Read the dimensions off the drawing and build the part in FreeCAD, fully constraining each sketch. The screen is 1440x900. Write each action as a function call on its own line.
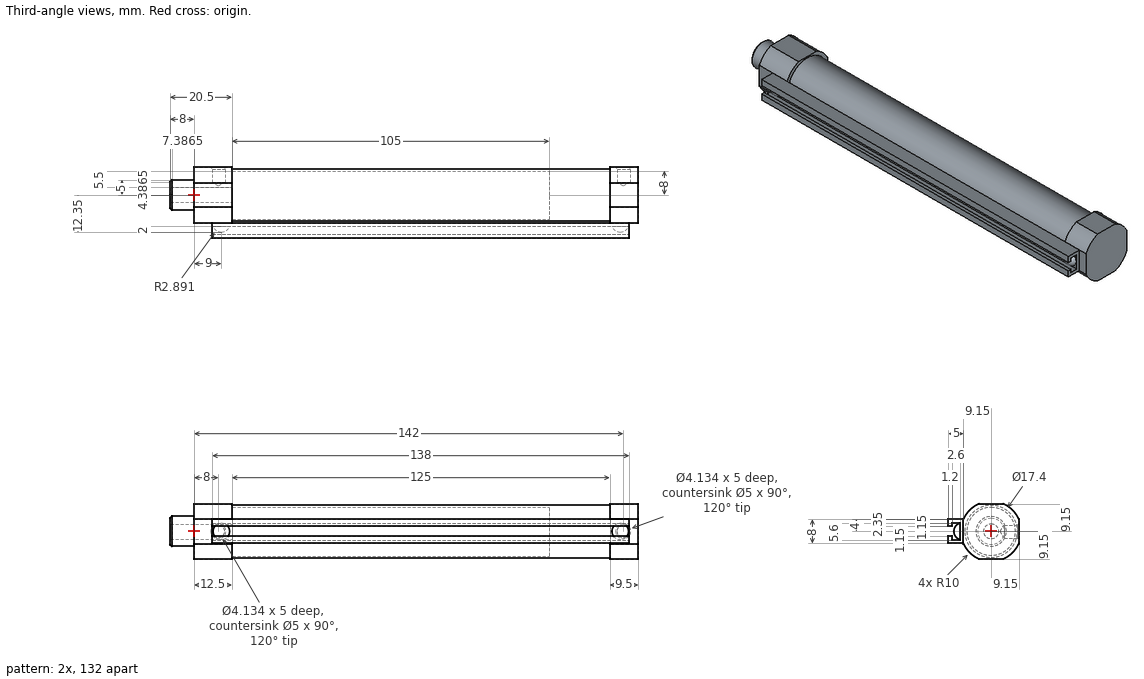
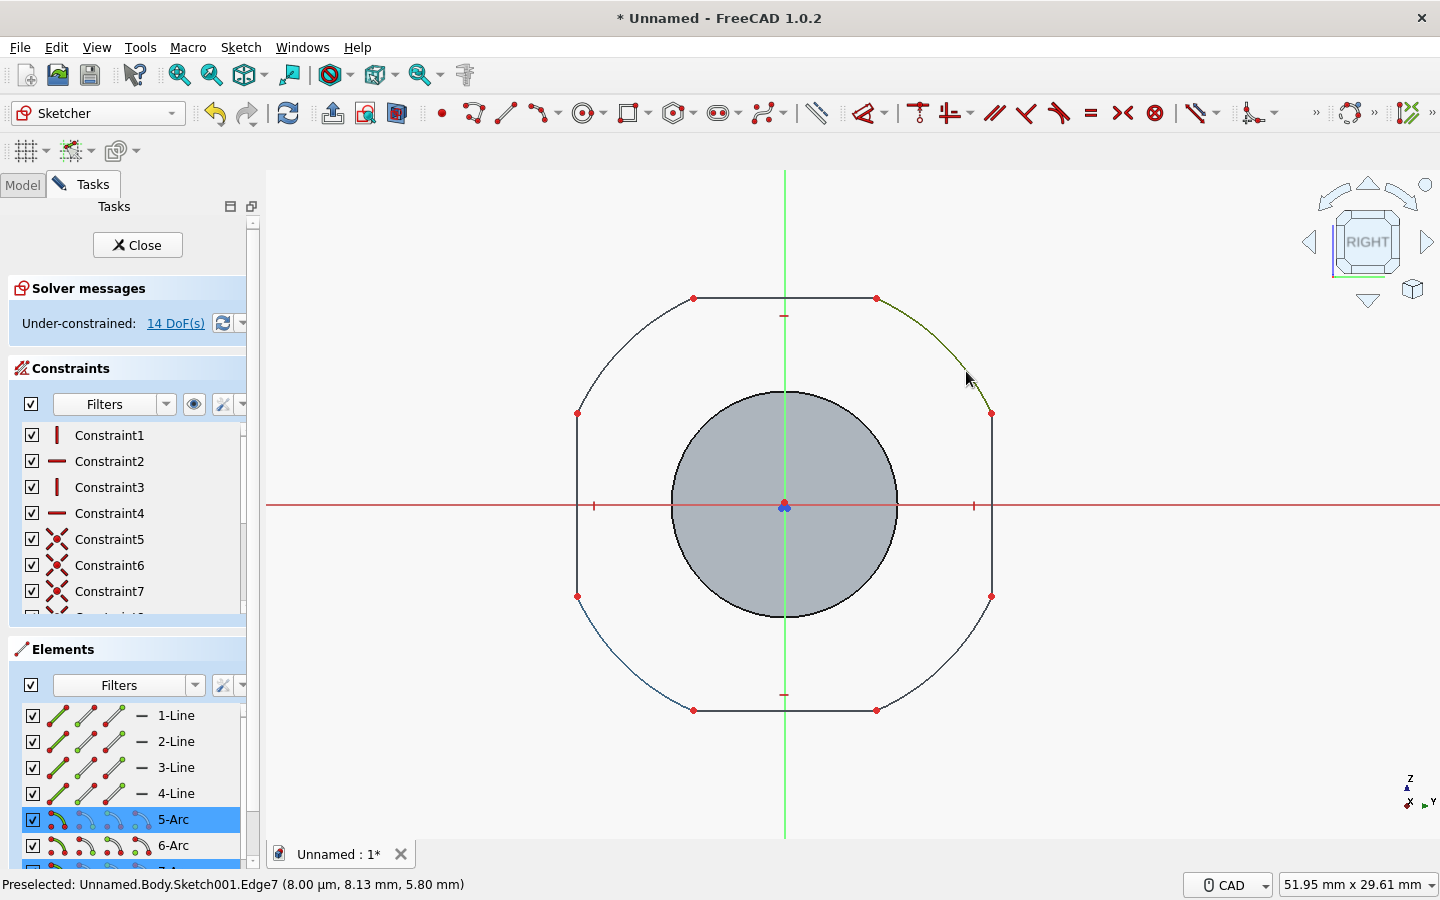
click(918, 114)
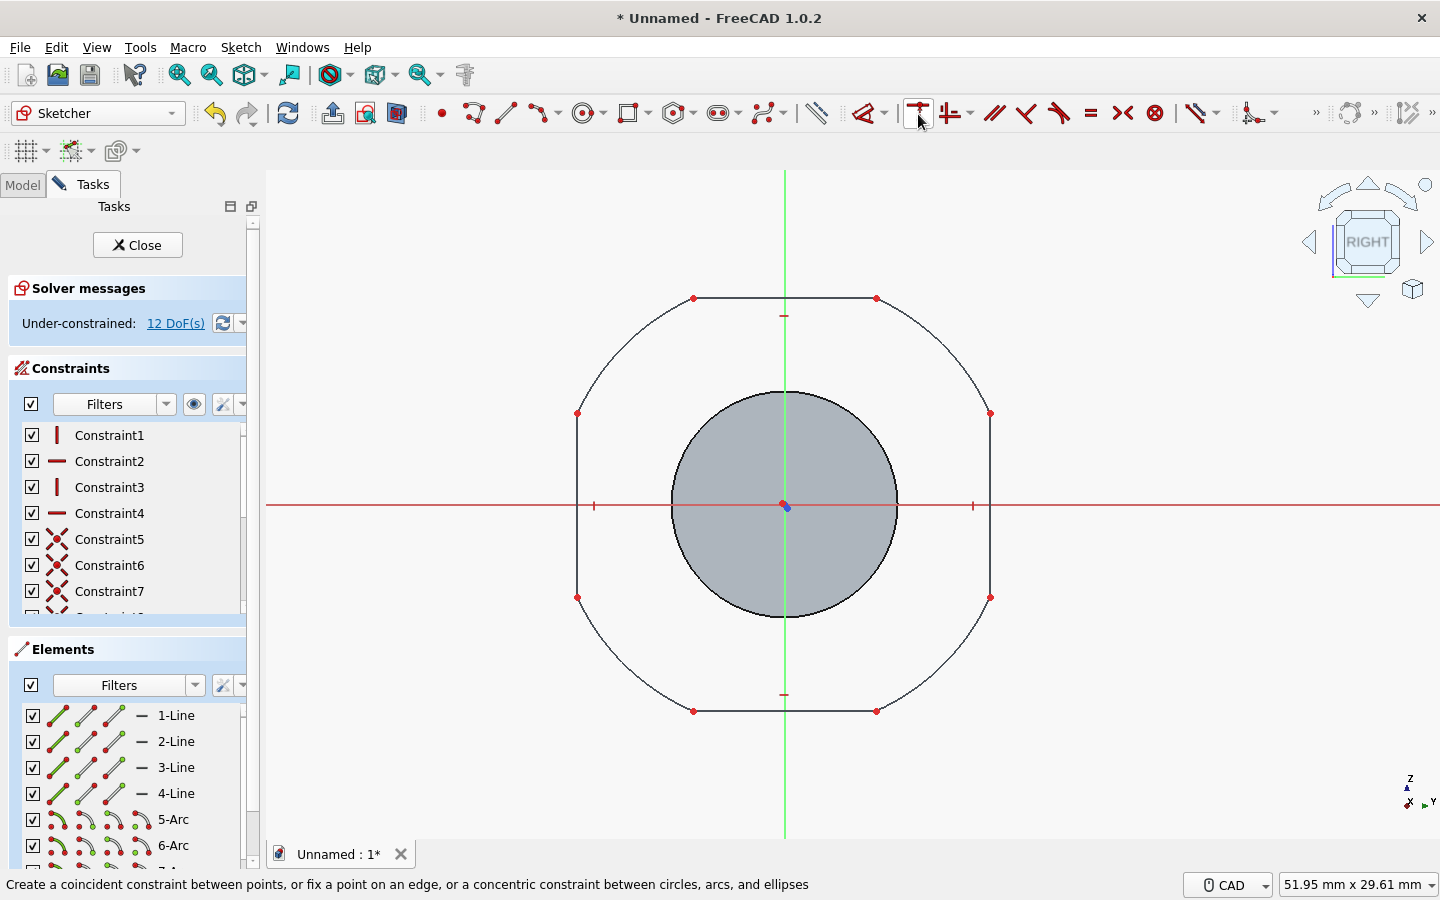
click(603, 640)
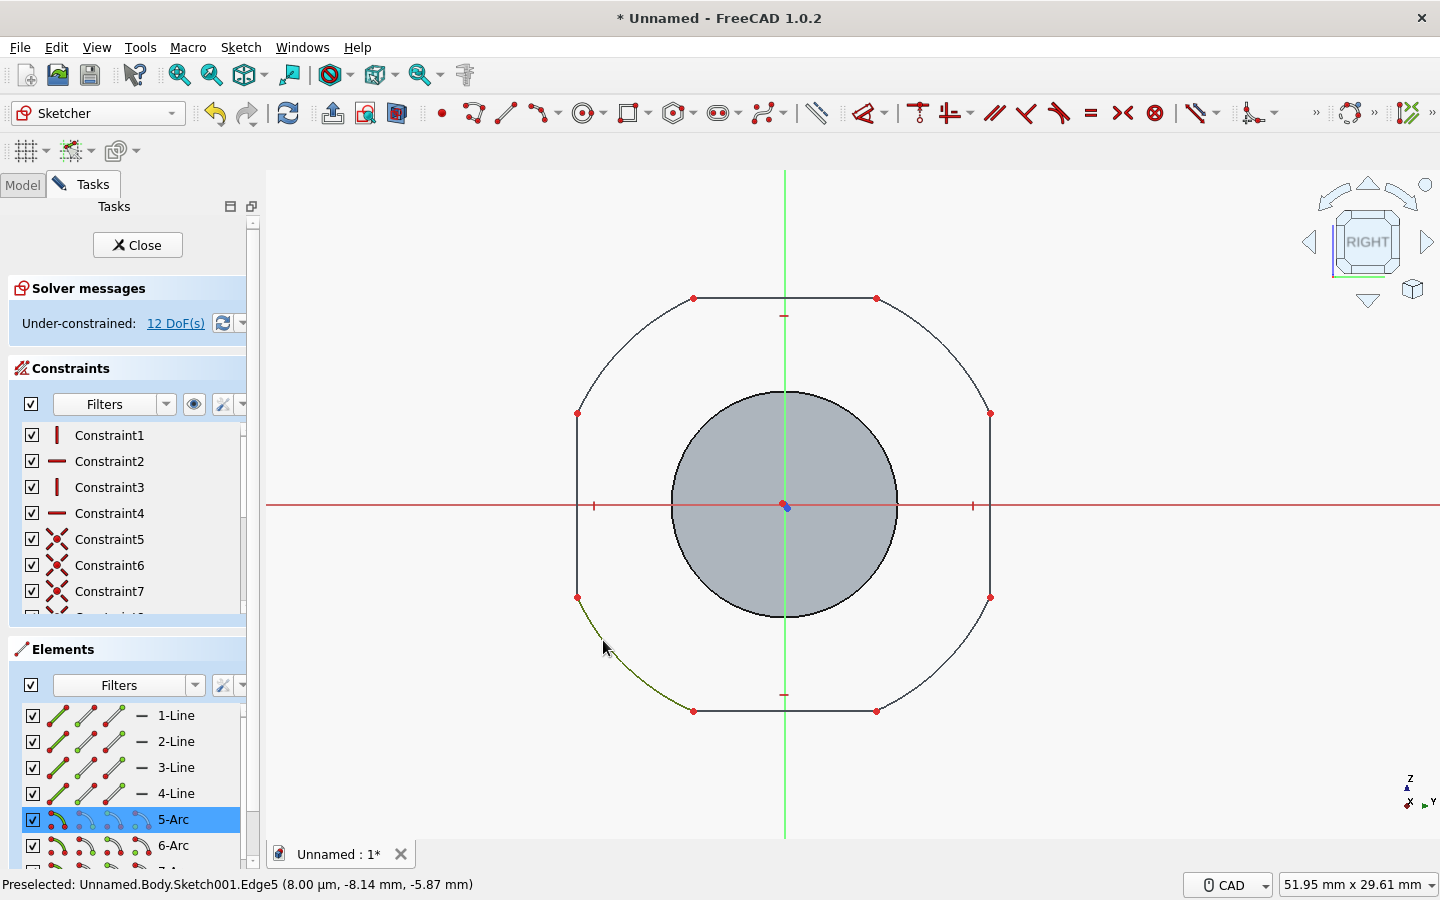
click(650, 324)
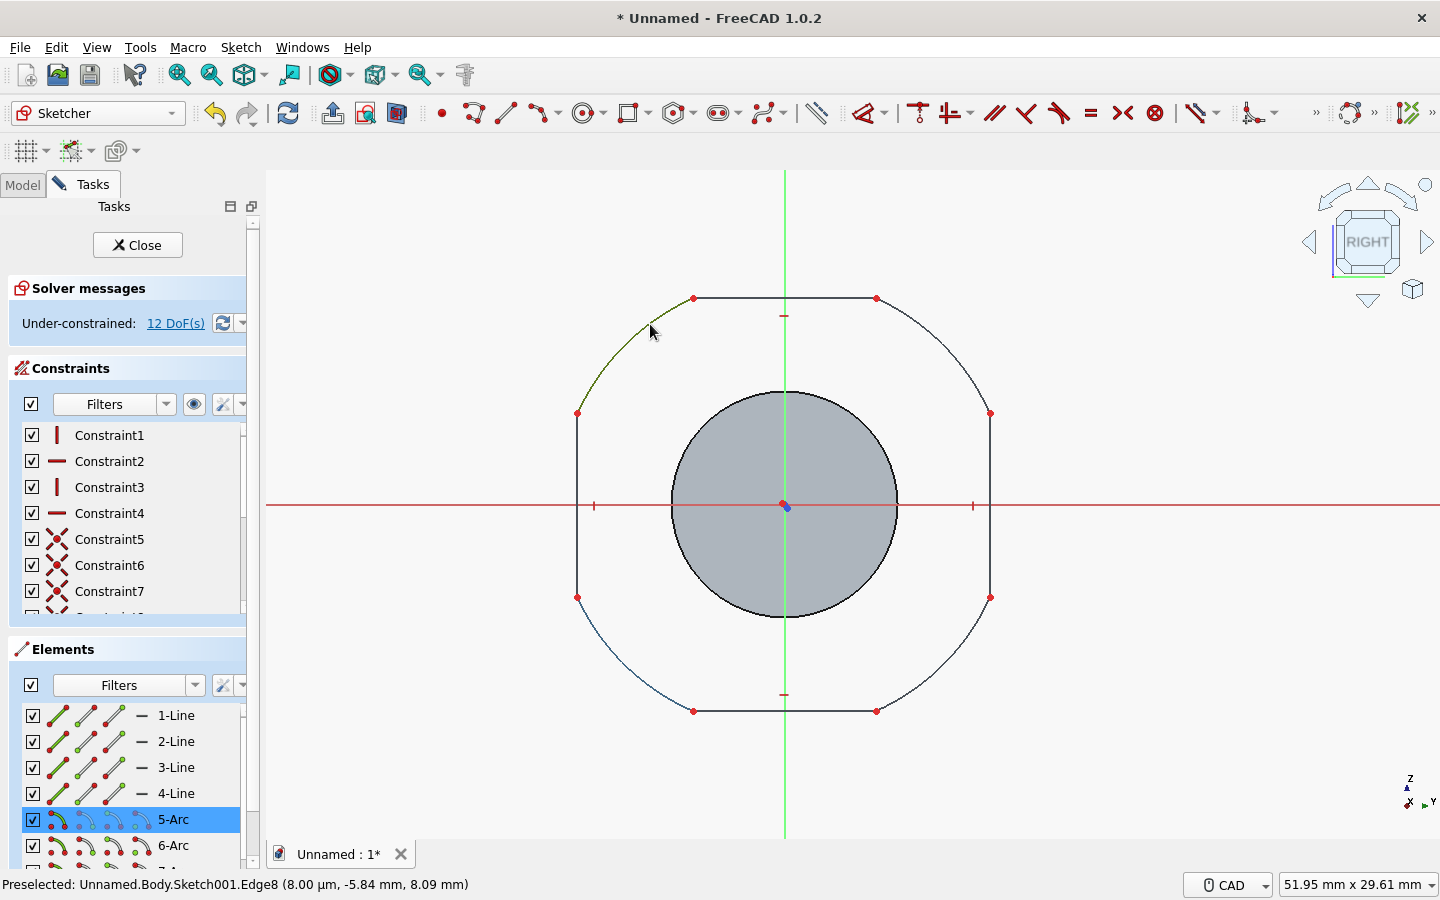
click(918, 114)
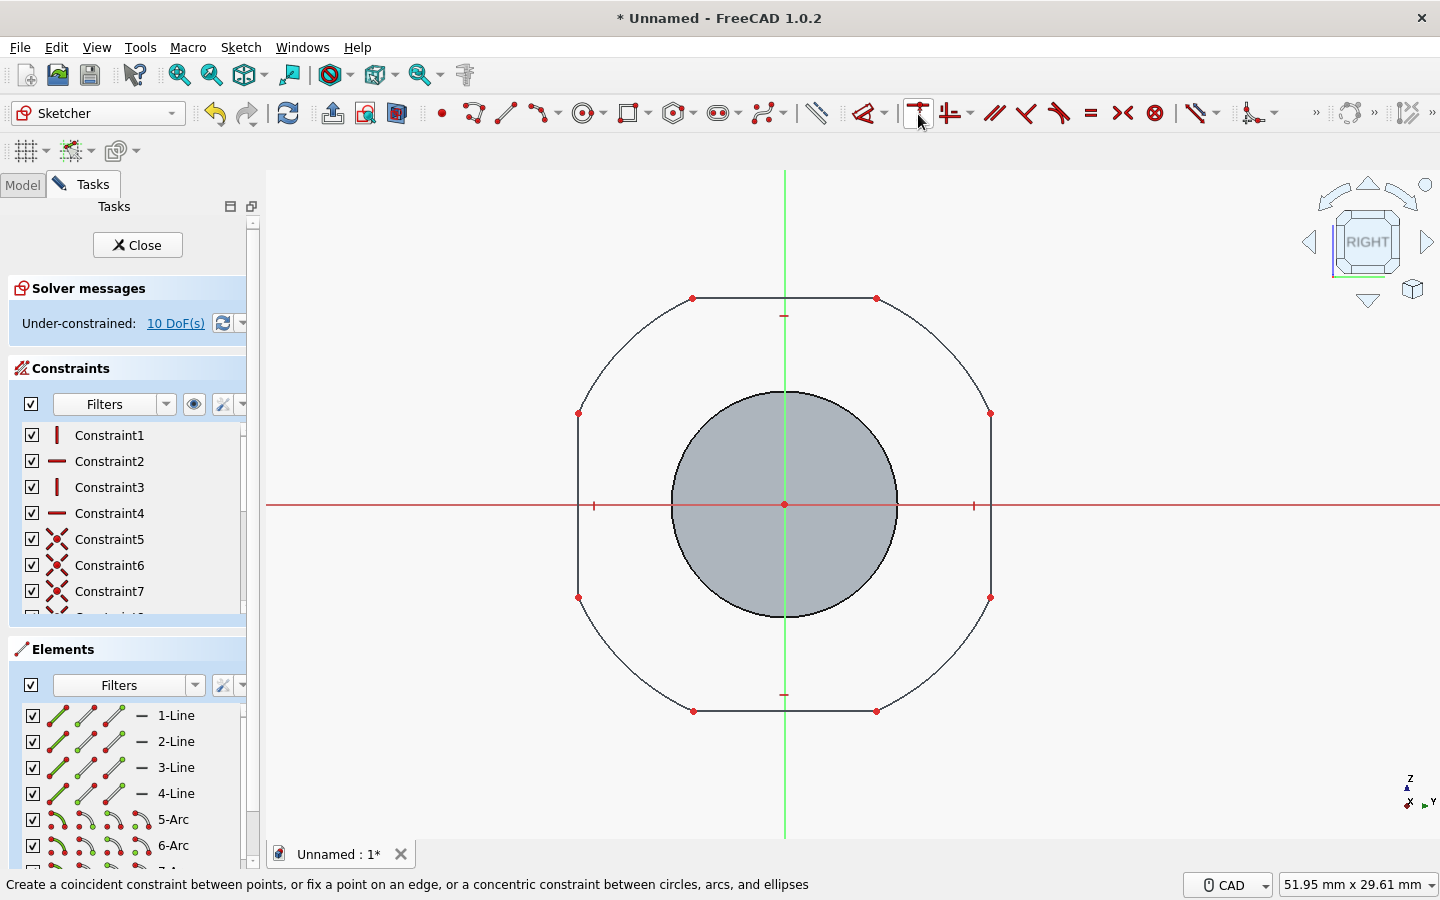
drag(774, 494, 795, 514)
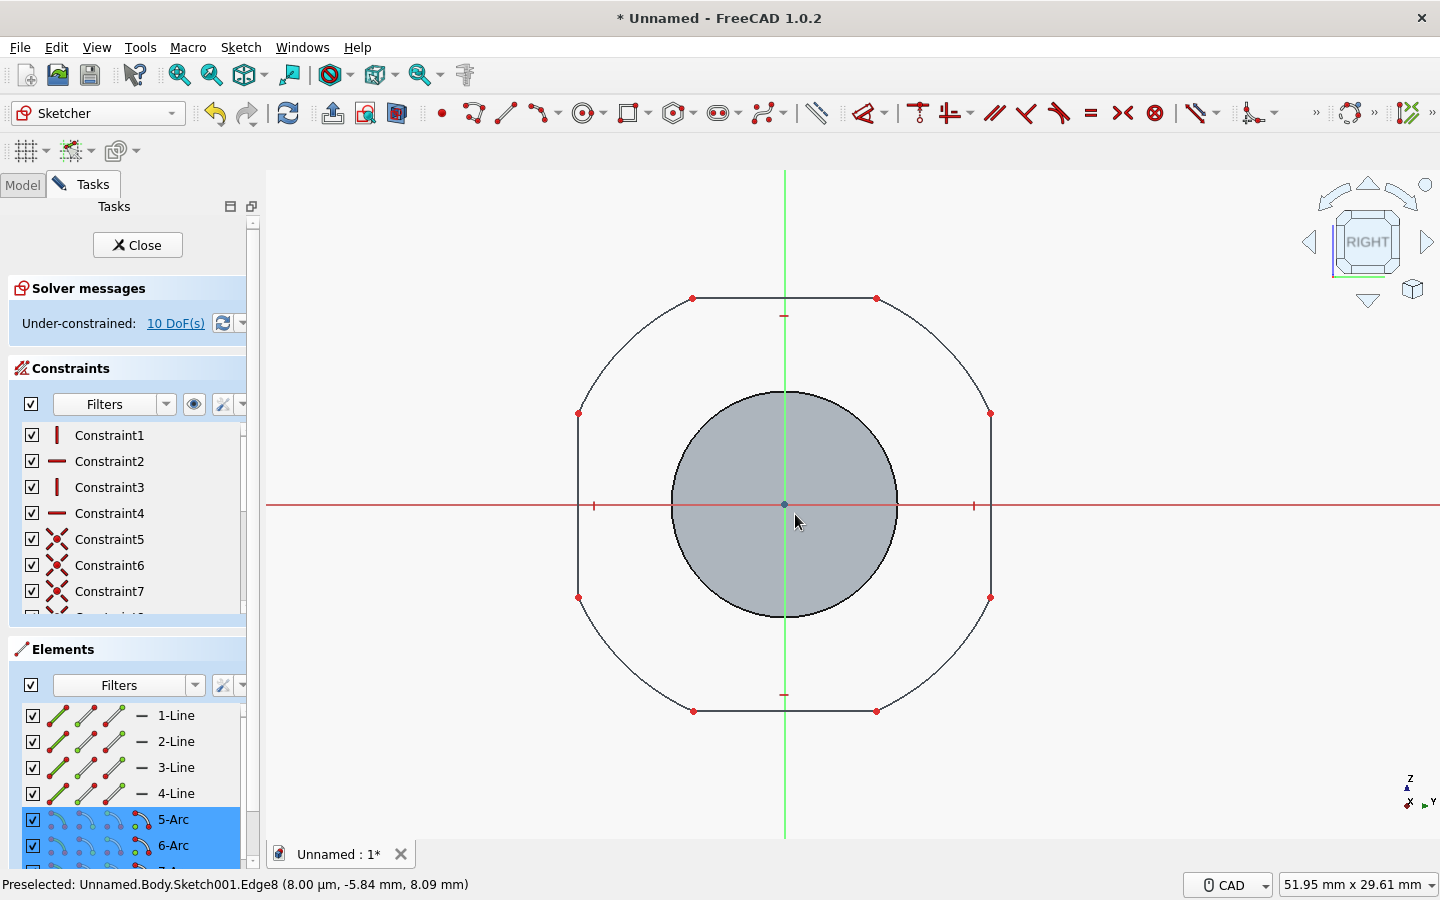
click(918, 114)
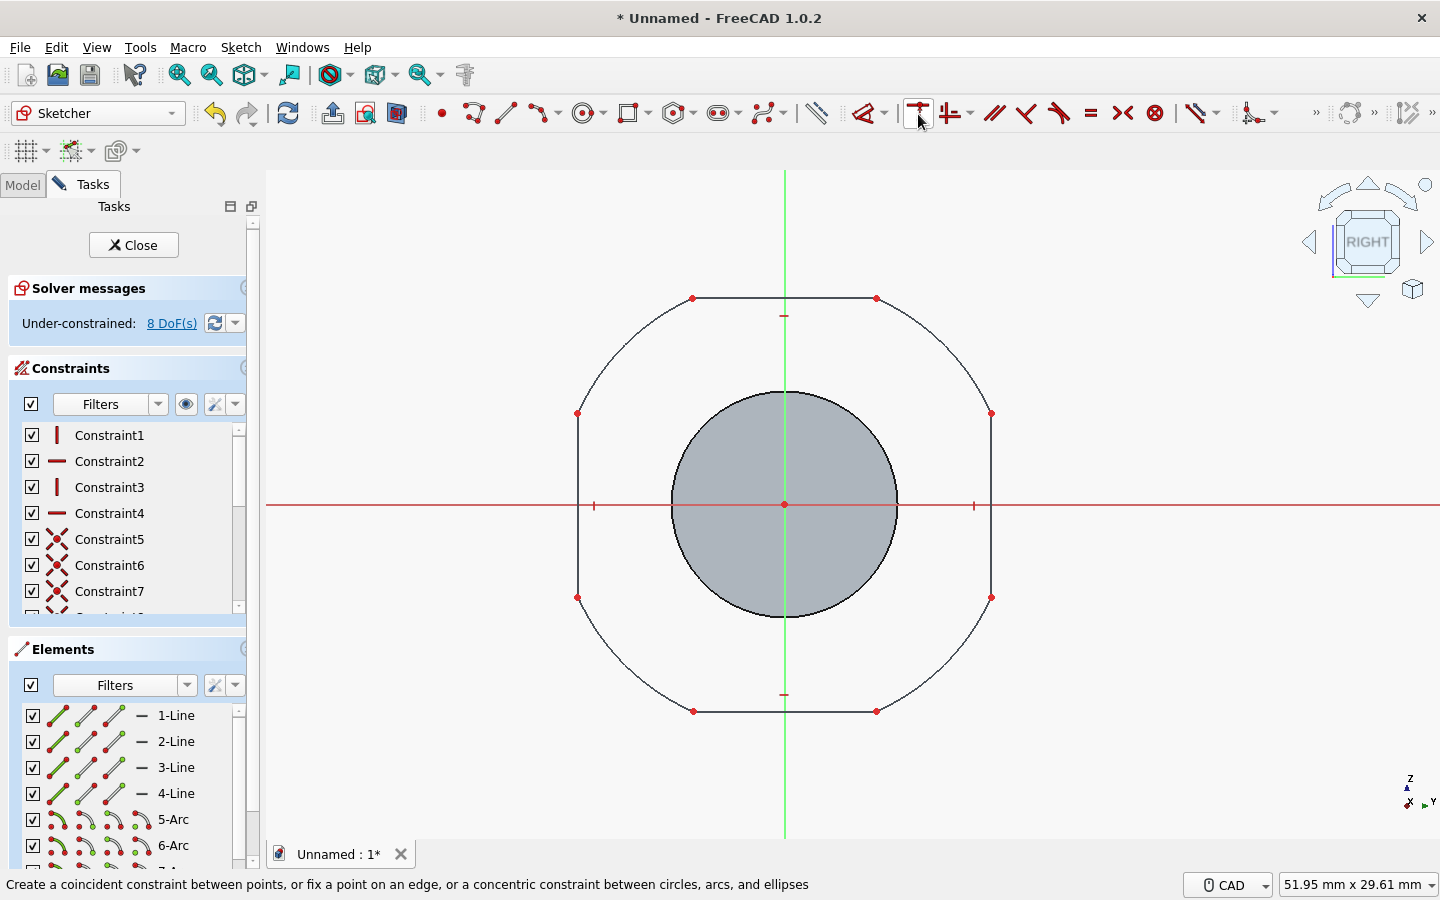
click(603, 640)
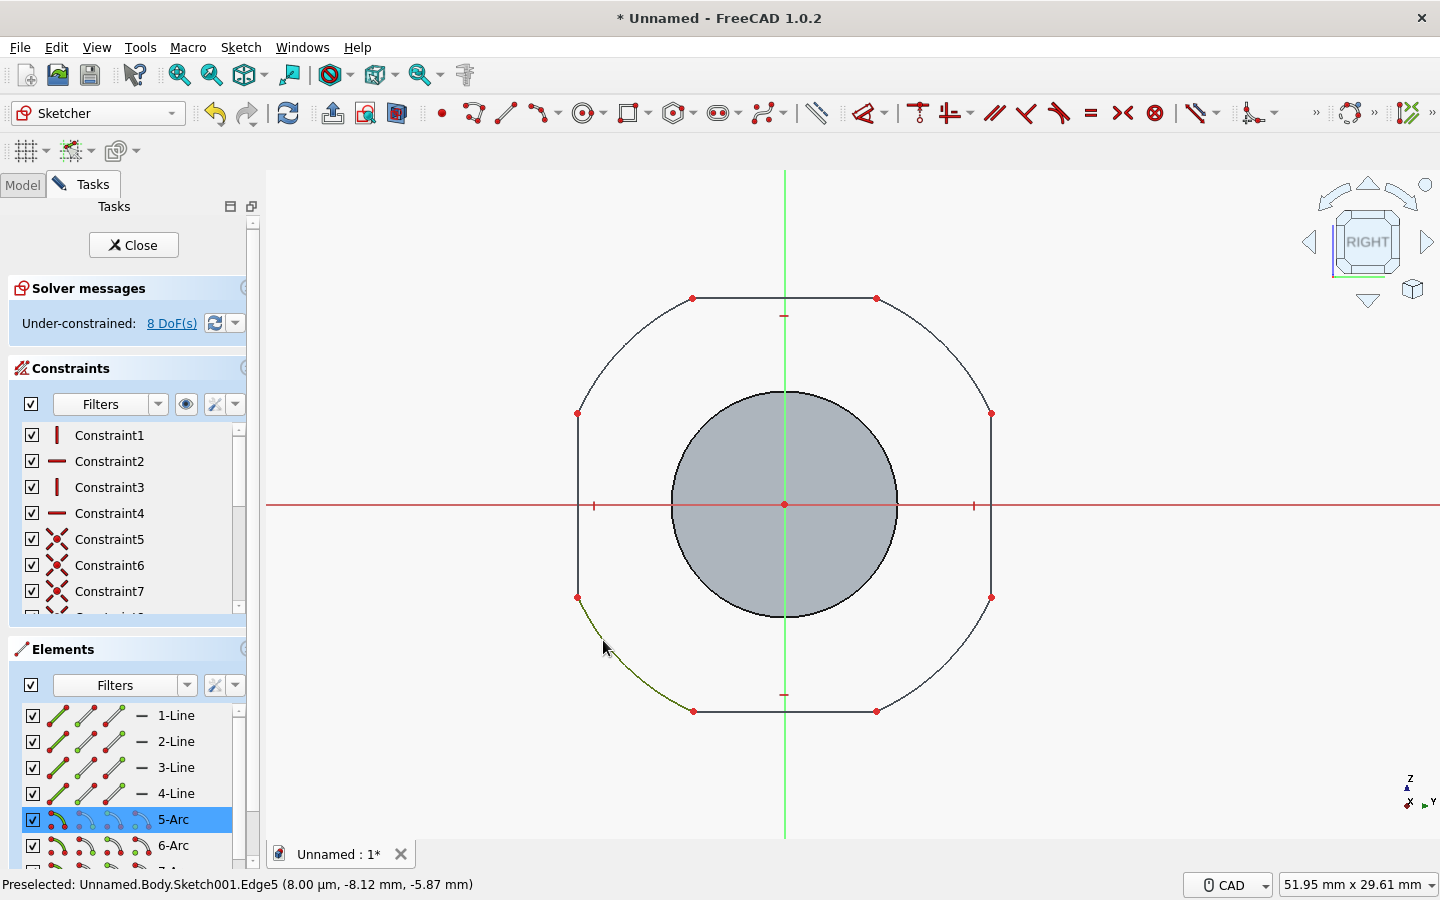
click(919, 687)